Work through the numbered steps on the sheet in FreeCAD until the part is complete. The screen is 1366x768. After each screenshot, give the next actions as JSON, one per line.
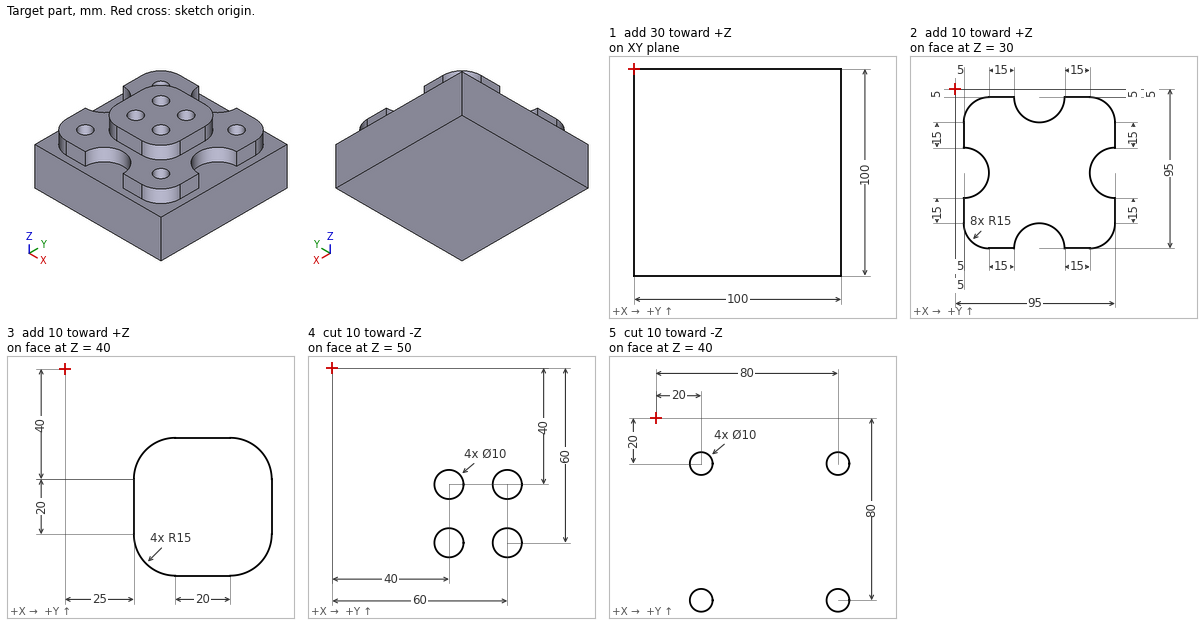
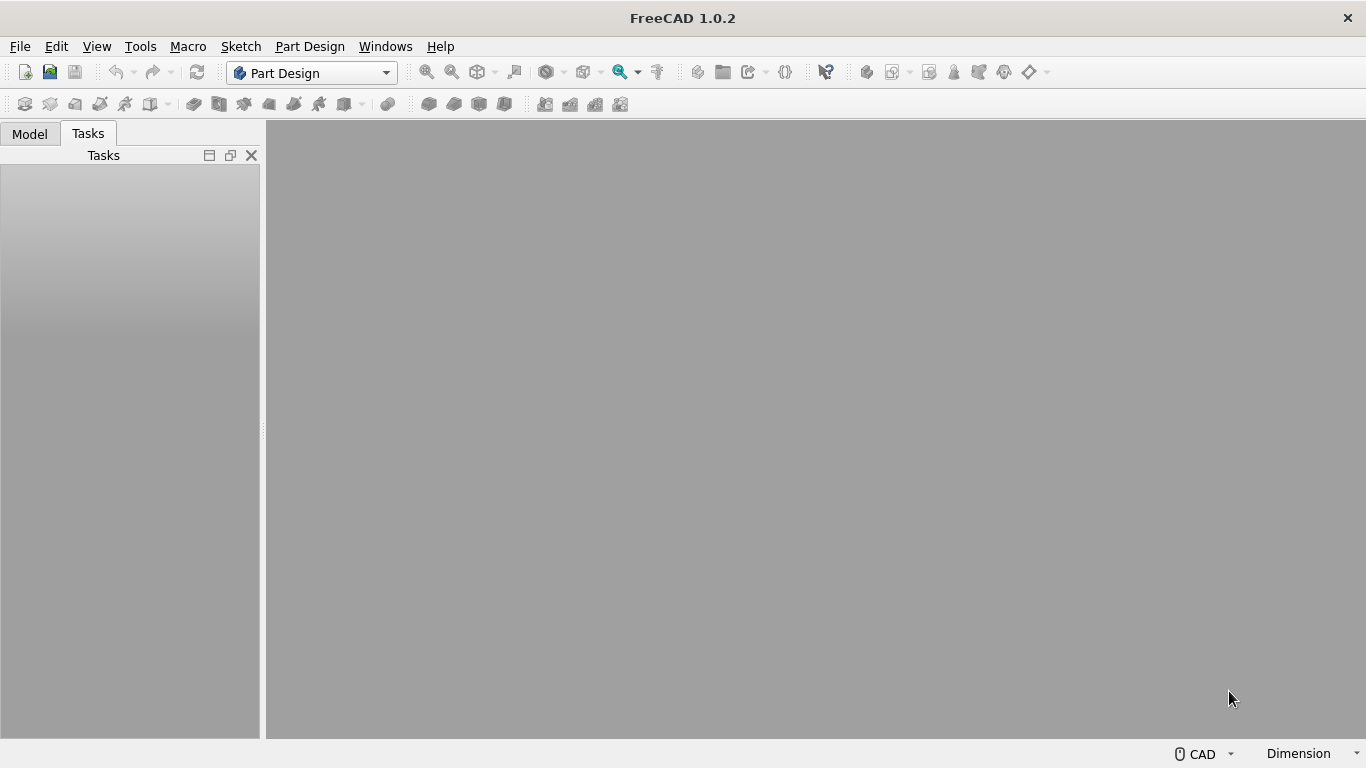
{"action": "left_click", "coordinate": [25, 72]}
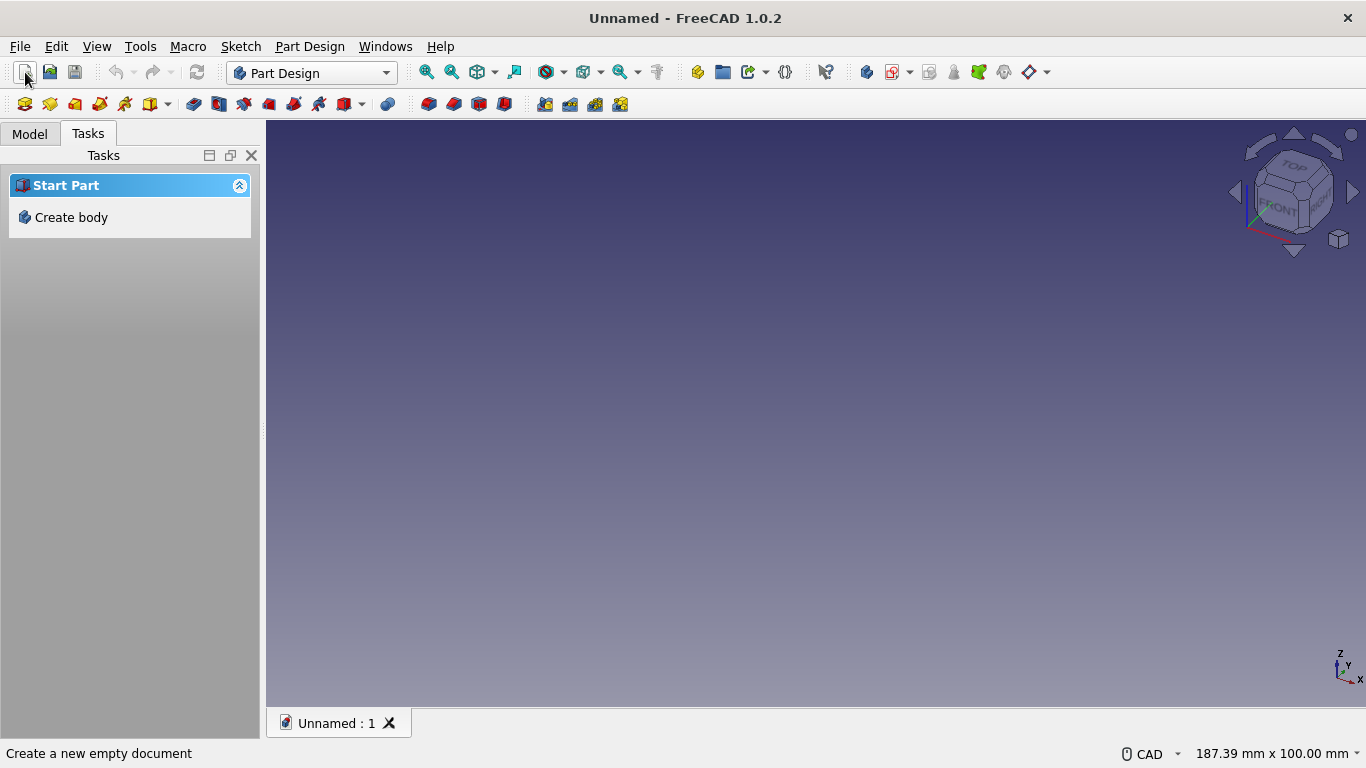
{"action": "left_click", "coordinate": [892, 72]}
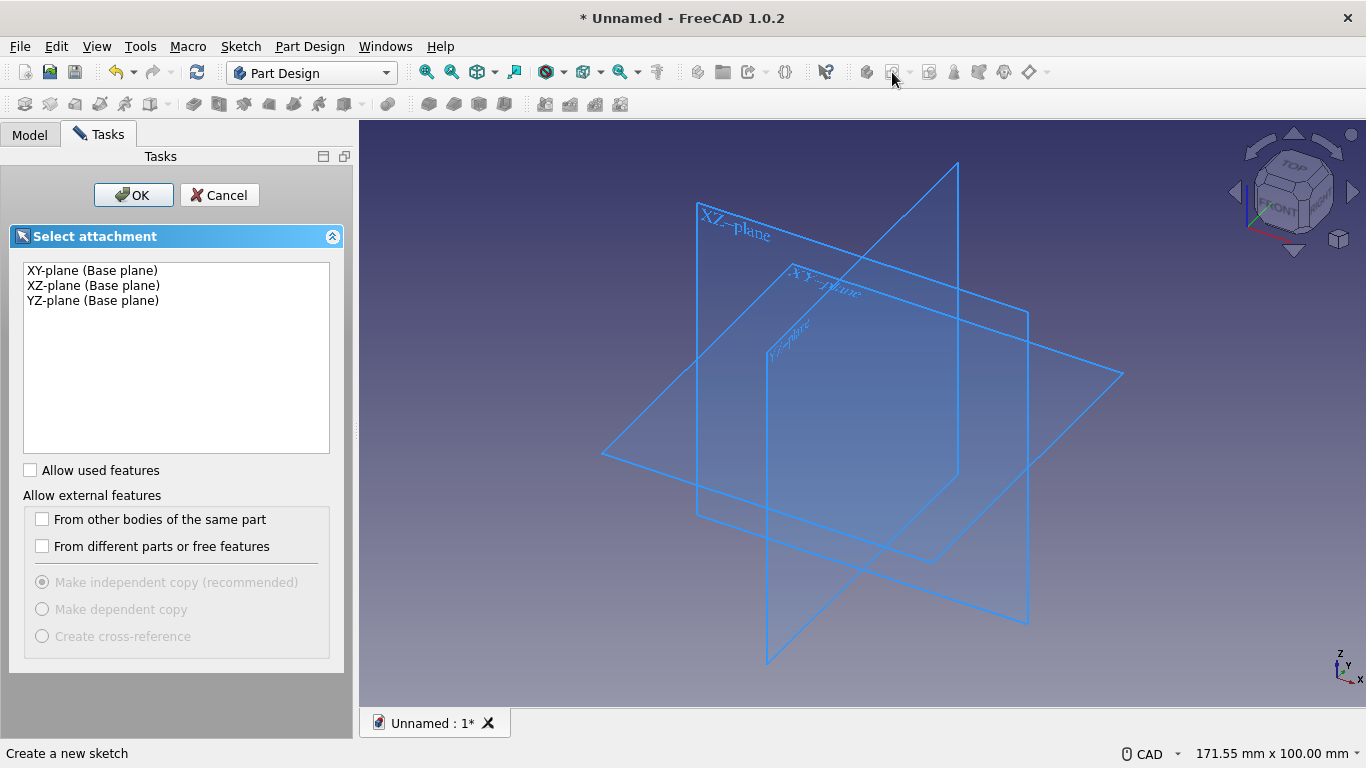
{"action": "left_click", "coordinate": [84, 270]}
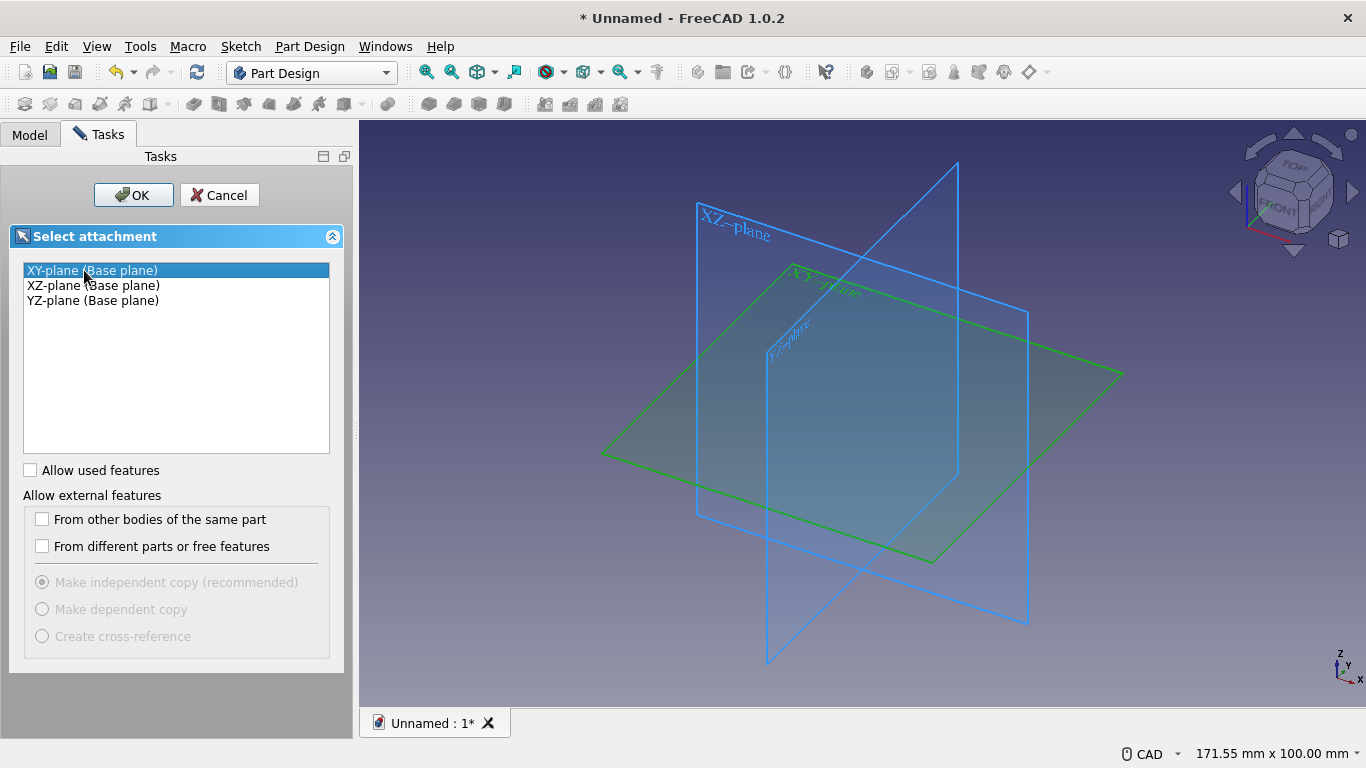
{"action": "left_click", "coordinate": [134, 195]}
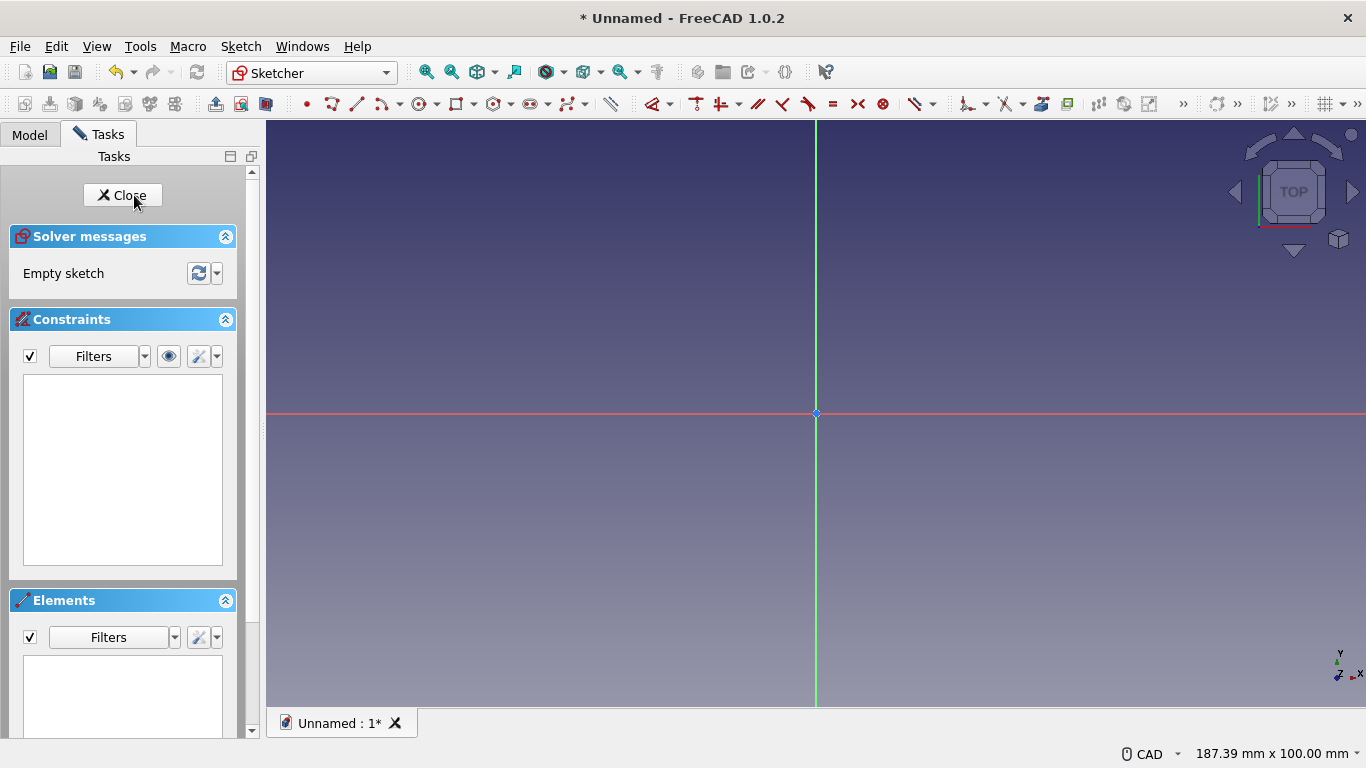
{"action": "scroll", "coordinate": [307, 148], "scroll_direction": "down", "scroll_amount": 3}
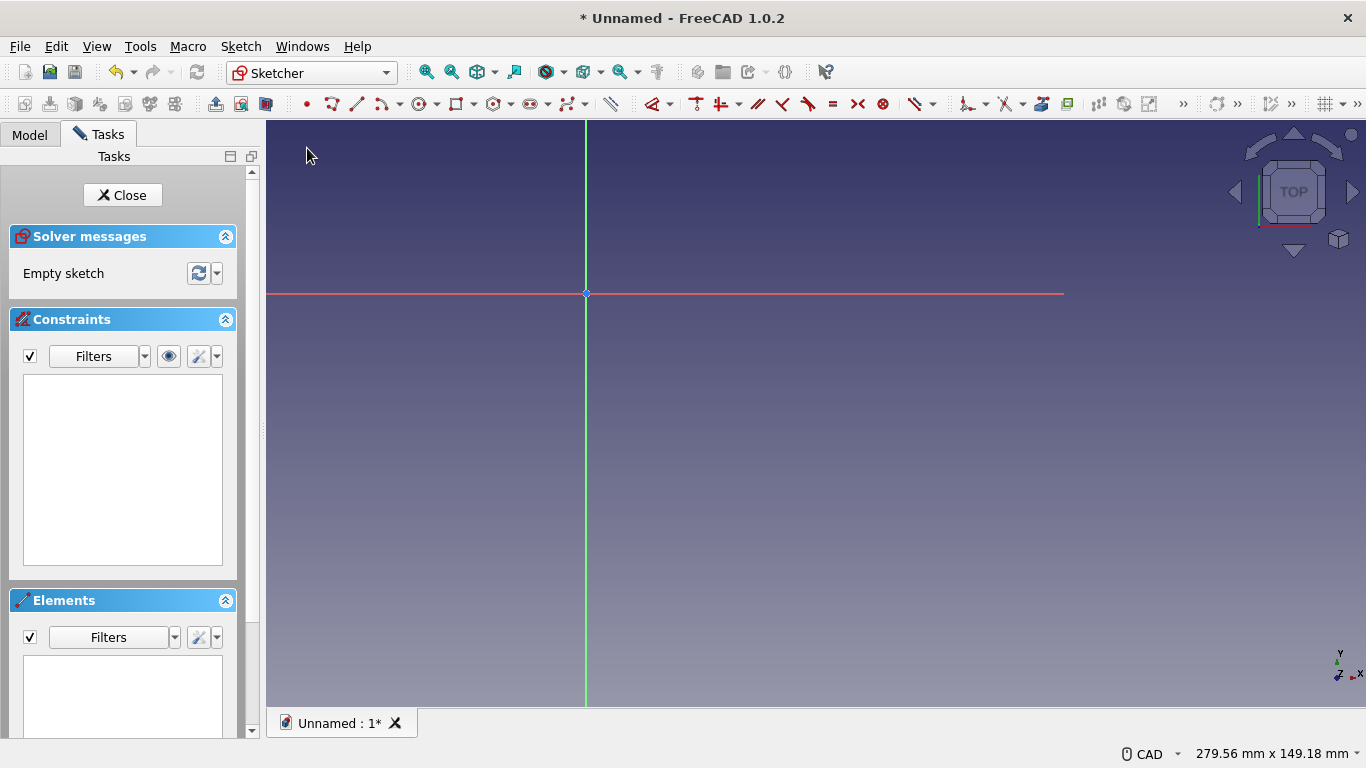
{"action": "left_click", "coordinate": [456, 104]}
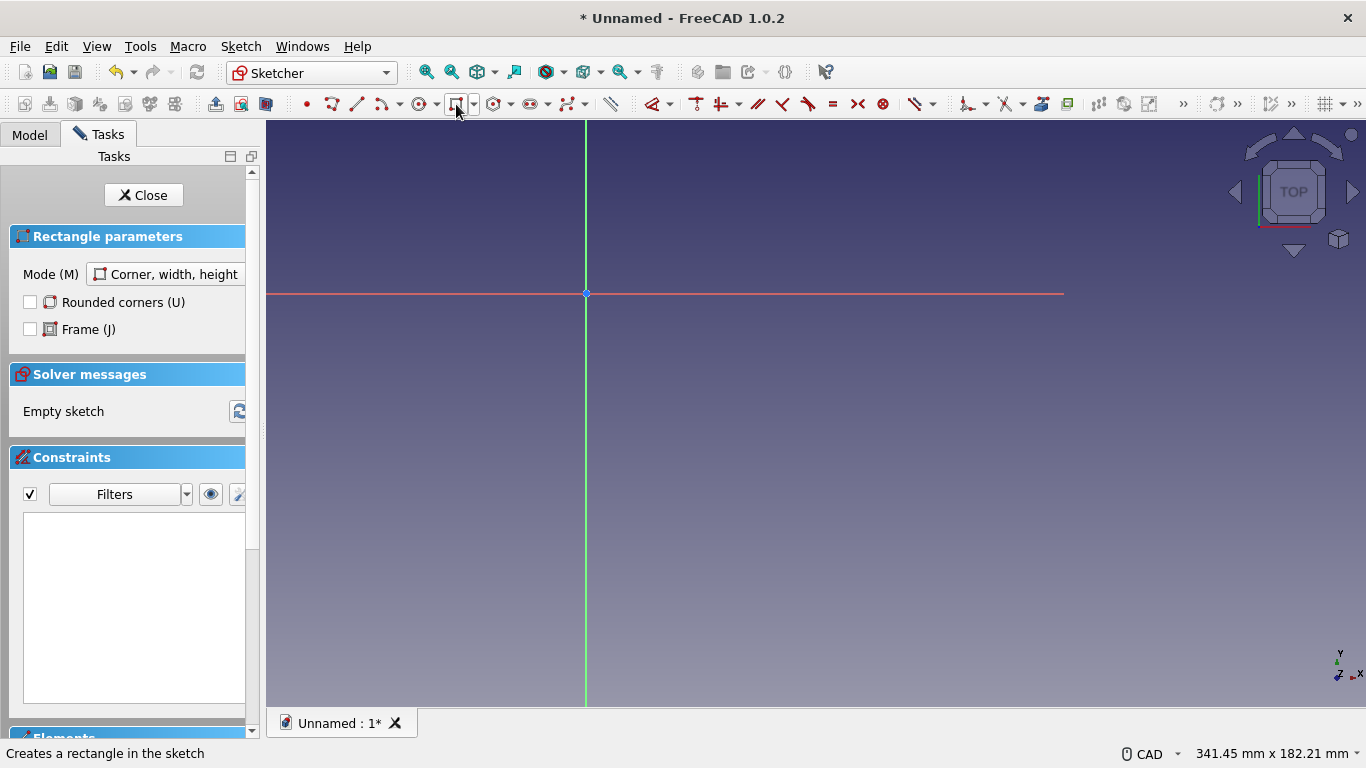
{"action": "left_click", "coordinate": [586, 294]}
{"action": "mouse_move", "coordinate": [909, 616]}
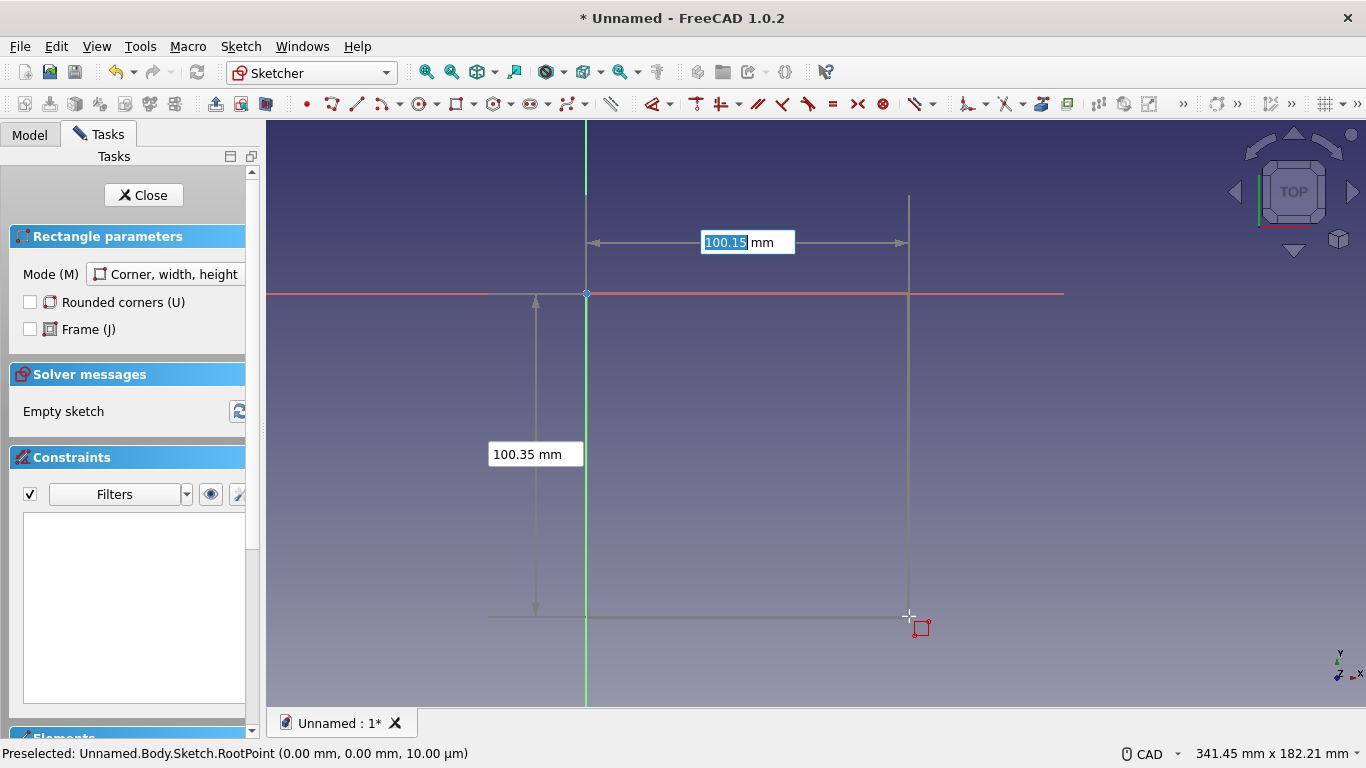
{"action": "type", "text": "100"}
{"action": "key", "text": "Tab"}
{"action": "type", "text": "100"}
{"action": "key", "text": "Return"}
{"action": "key", "text": "Escape"}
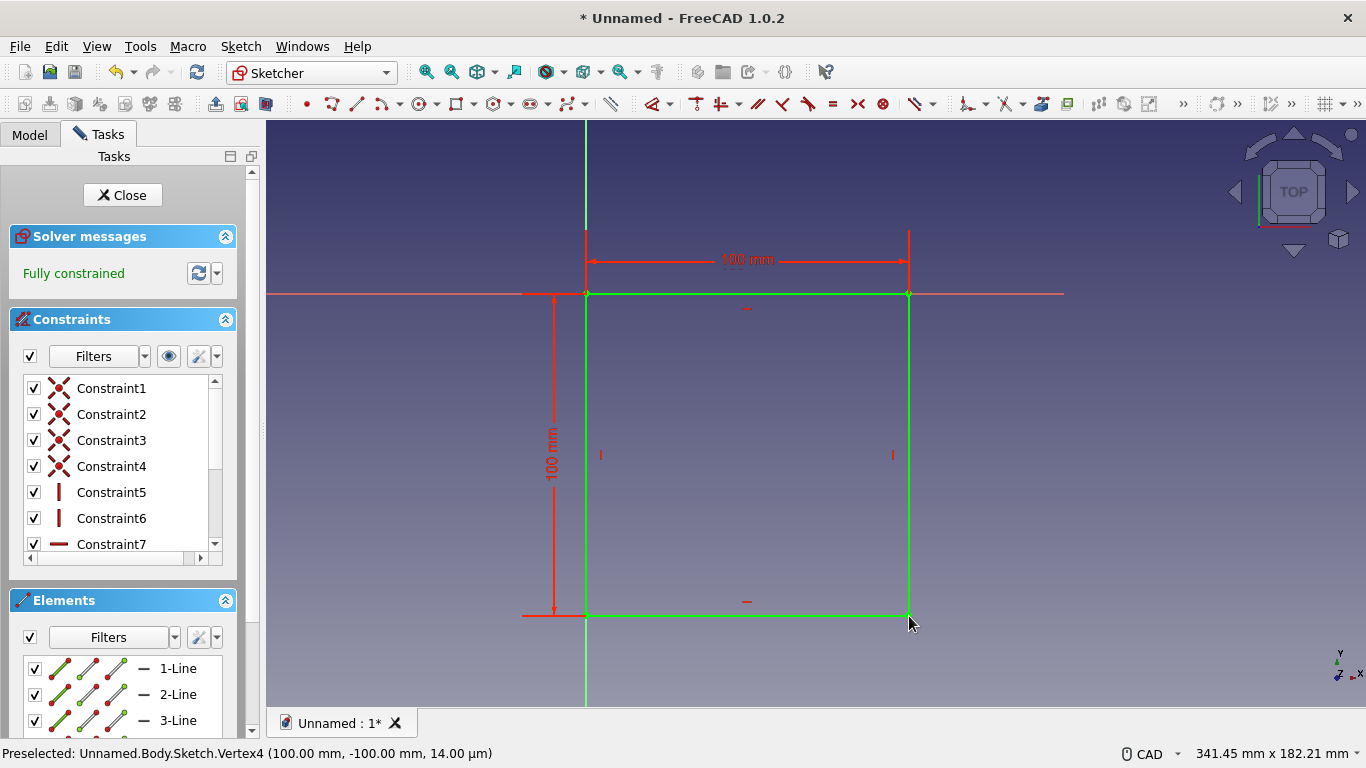
{"action": "left_click", "coordinate": [123, 195]}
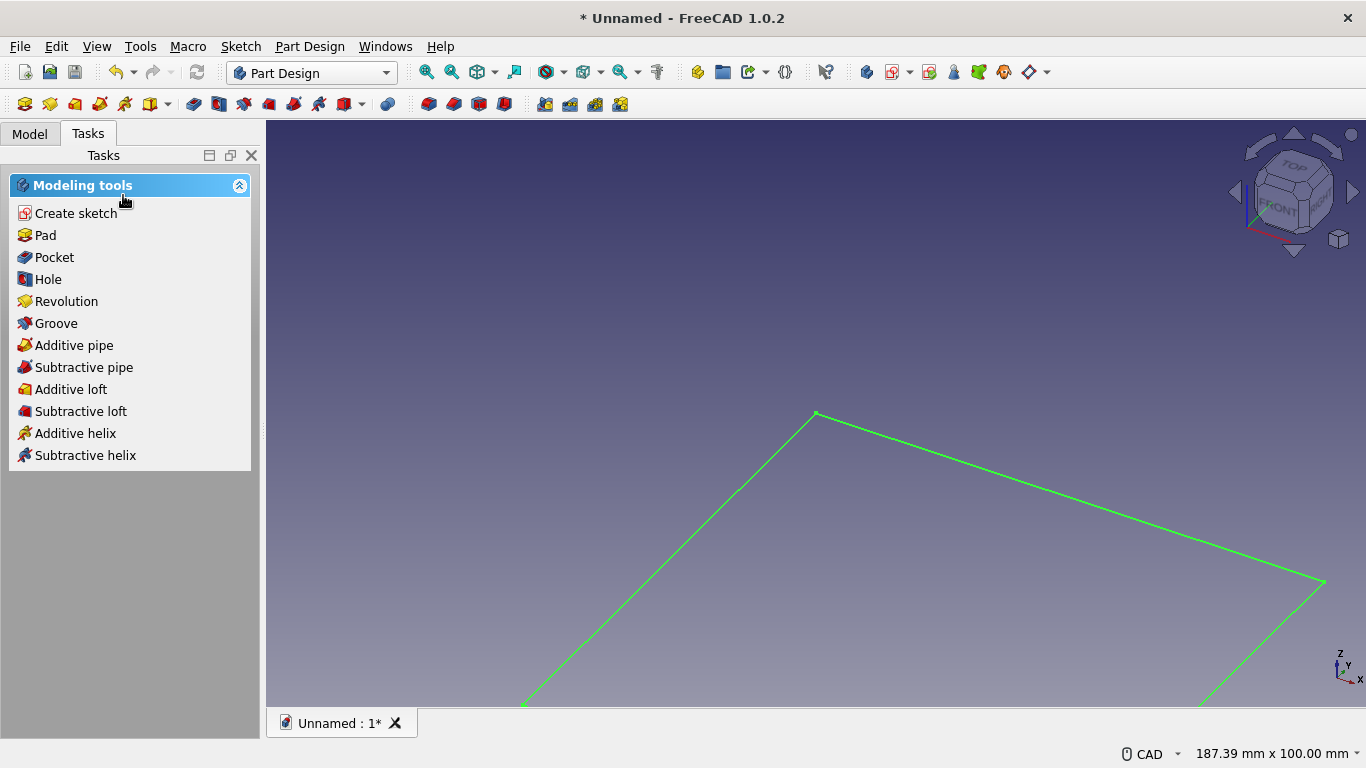
{"action": "left_click", "coordinate": [25, 104]}